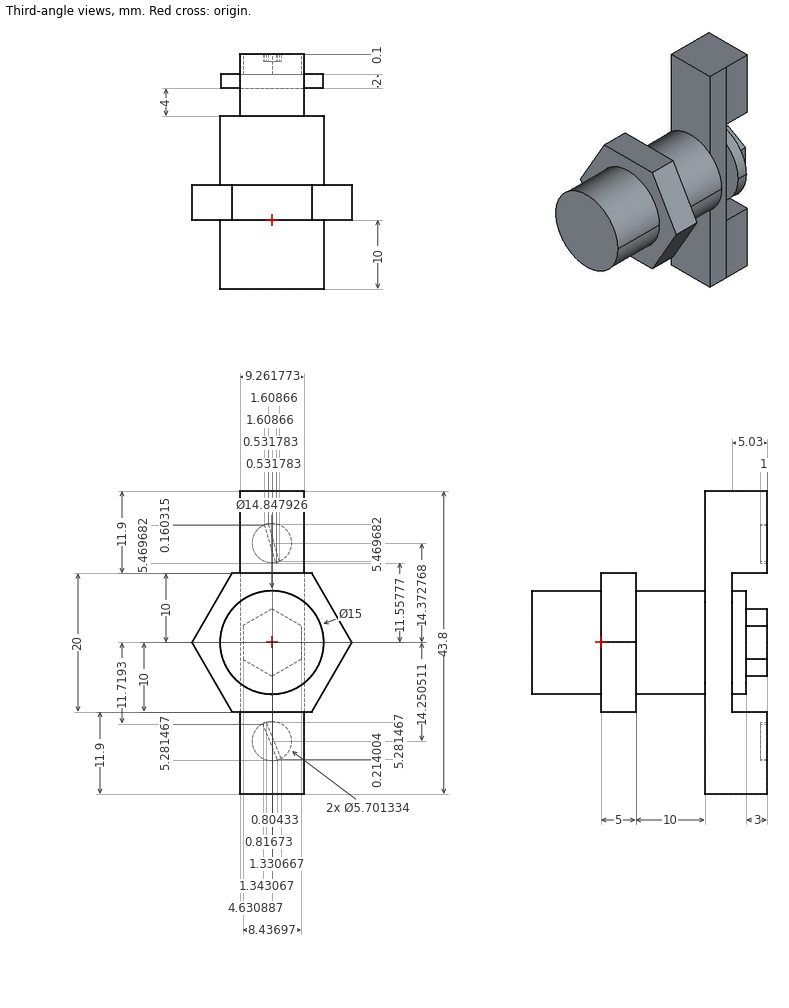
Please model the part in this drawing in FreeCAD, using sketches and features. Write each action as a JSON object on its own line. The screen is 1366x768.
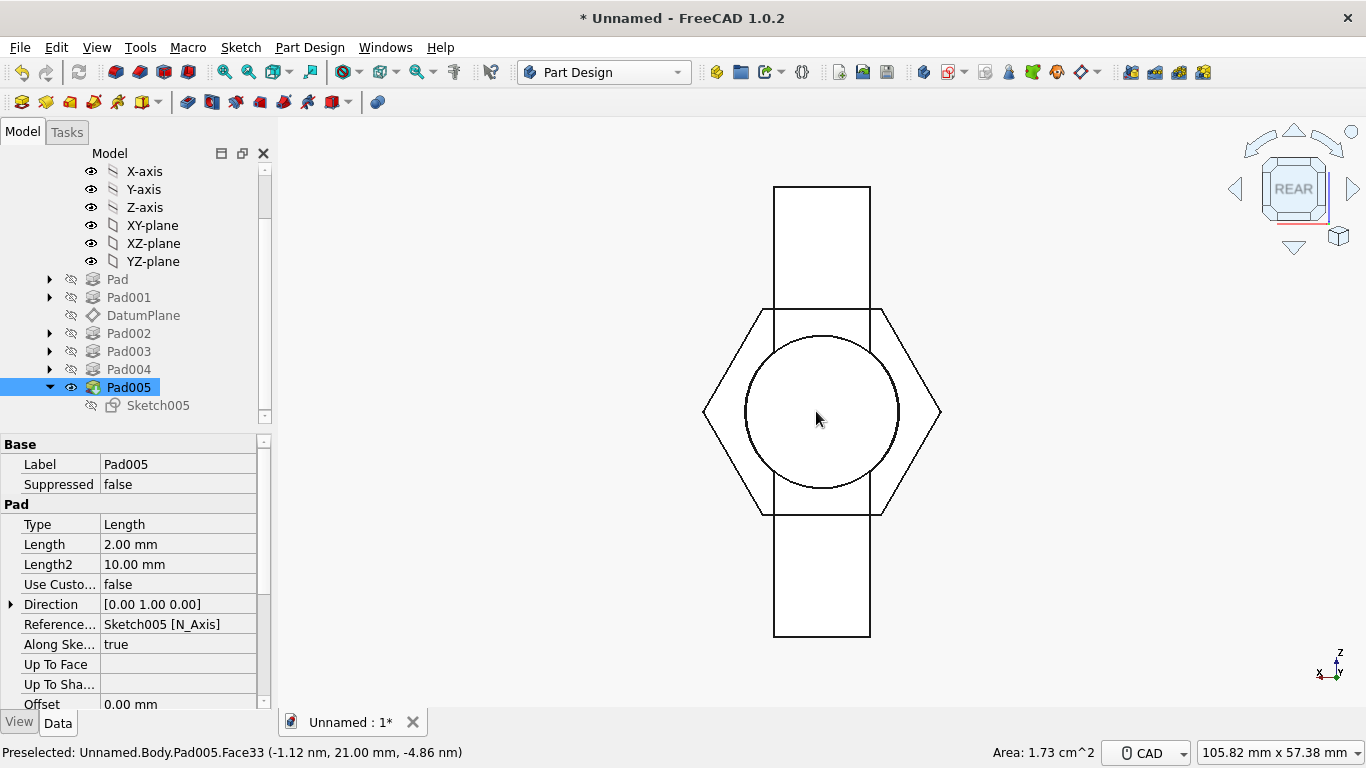
{"action": "left_click", "coordinate": [948, 72]}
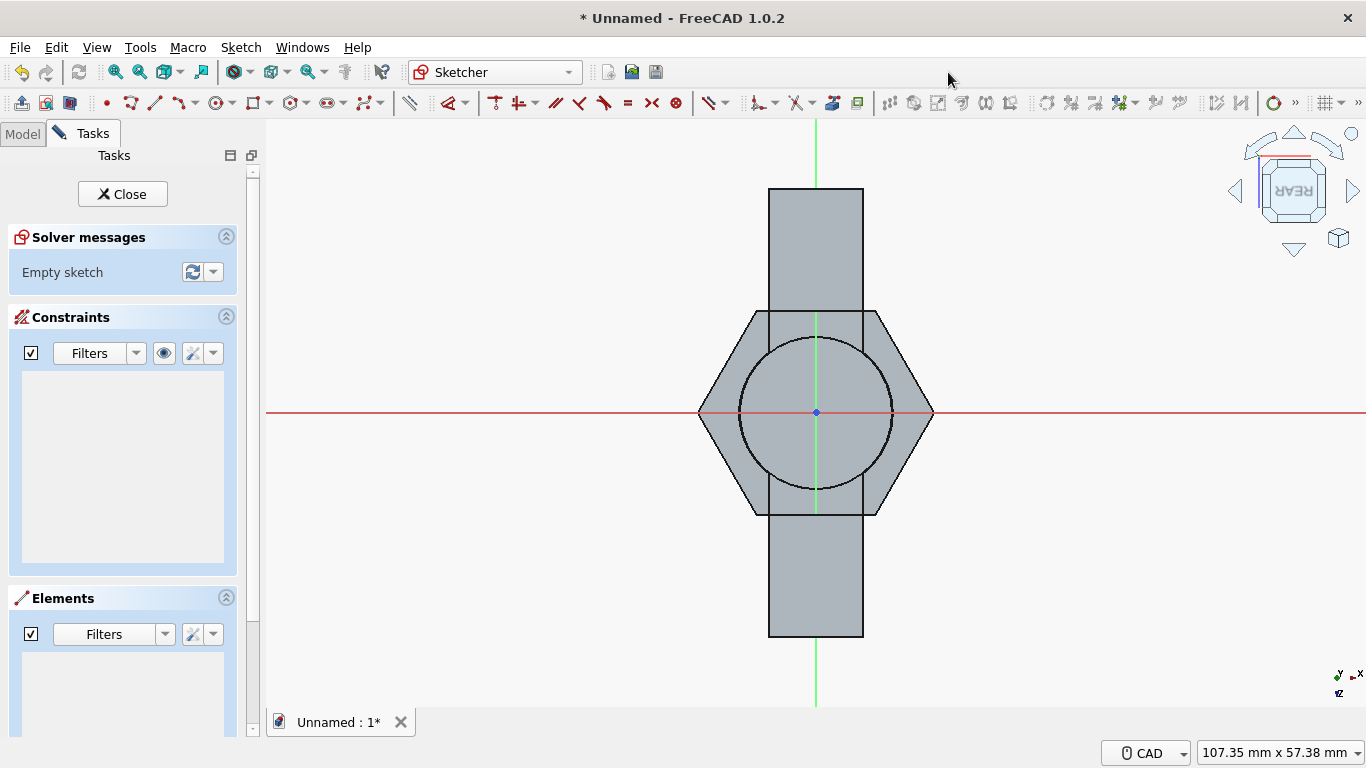
{"action": "scroll", "coordinate": [838, 413], "scroll_direction": "up", "scroll_amount": 7}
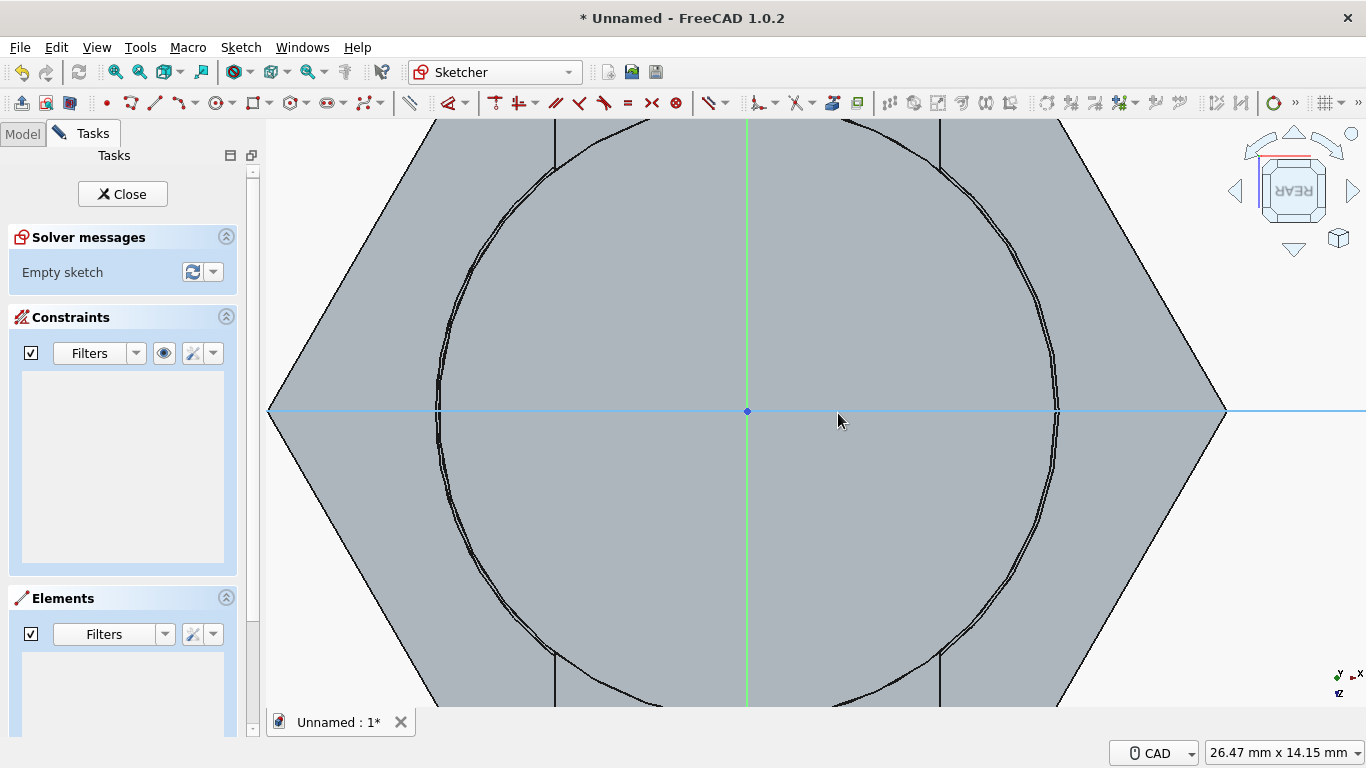
{"action": "left_click", "coordinate": [290, 104]}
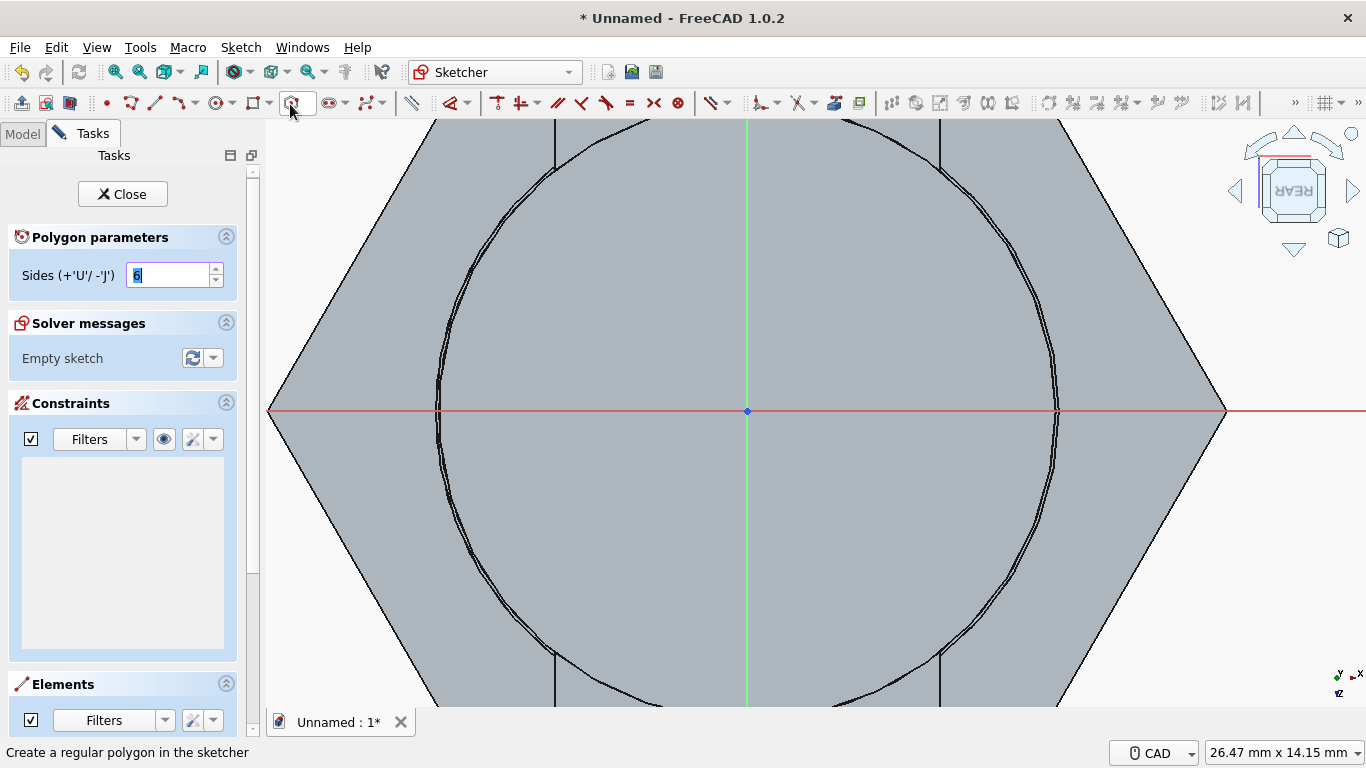
{"action": "left_click", "coordinate": [747, 411]}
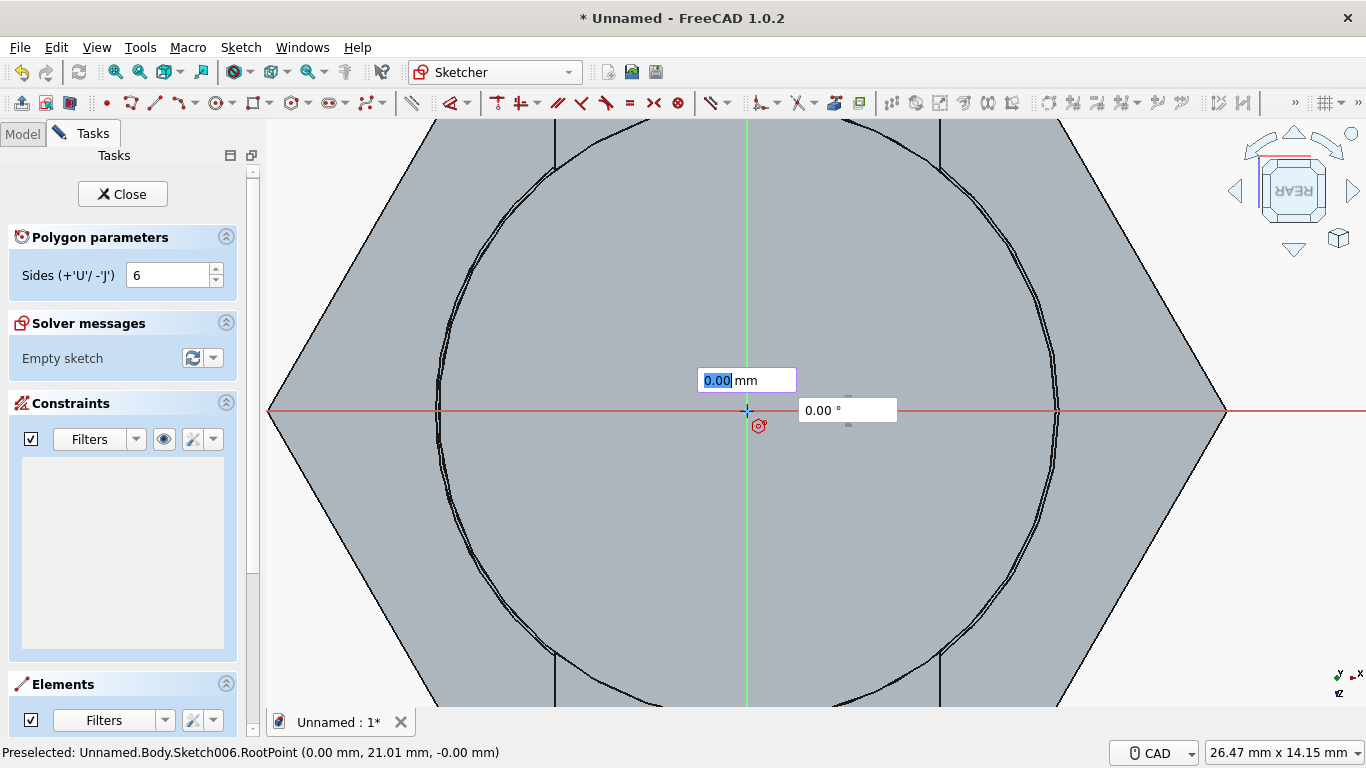
{"action": "left_click", "coordinate": [747, 209]}
{"action": "right_click", "coordinate": [747, 209]}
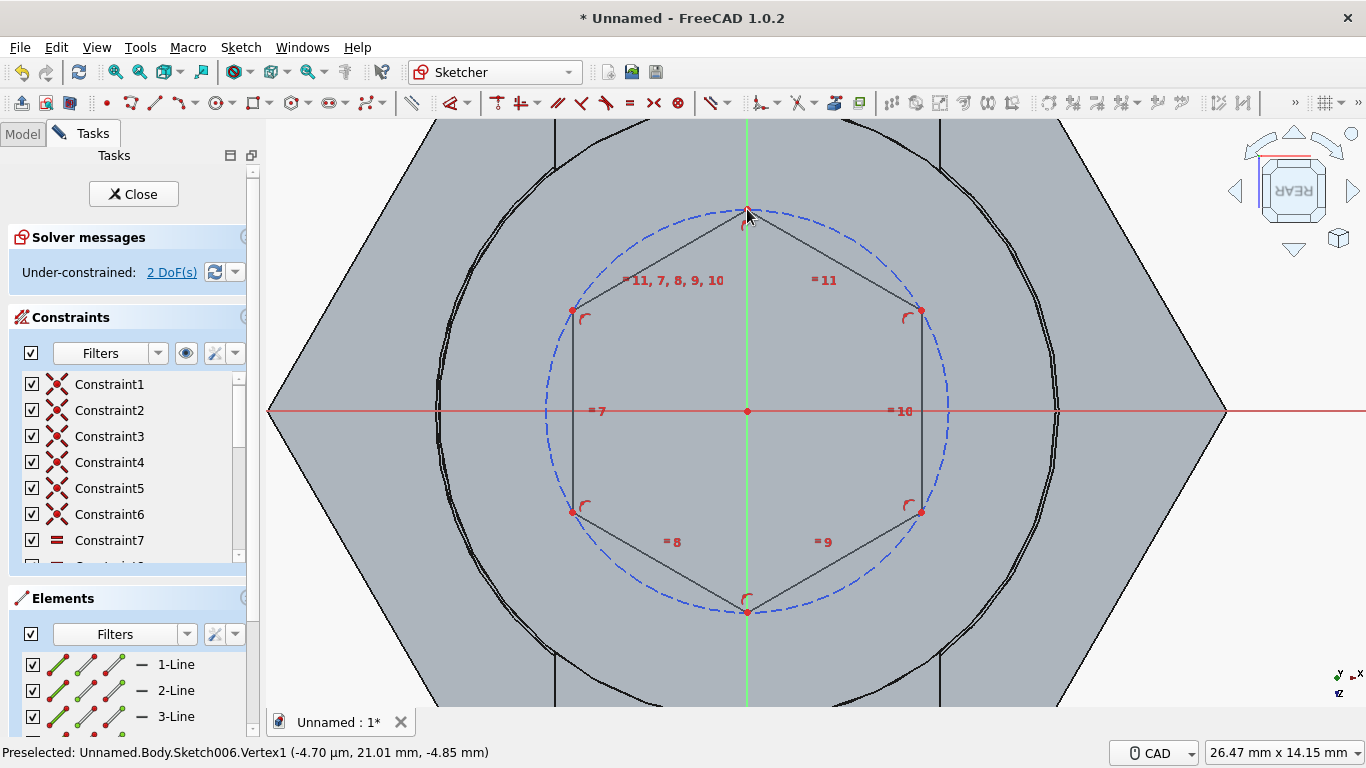
{"action": "left_click", "coordinate": [573, 371]}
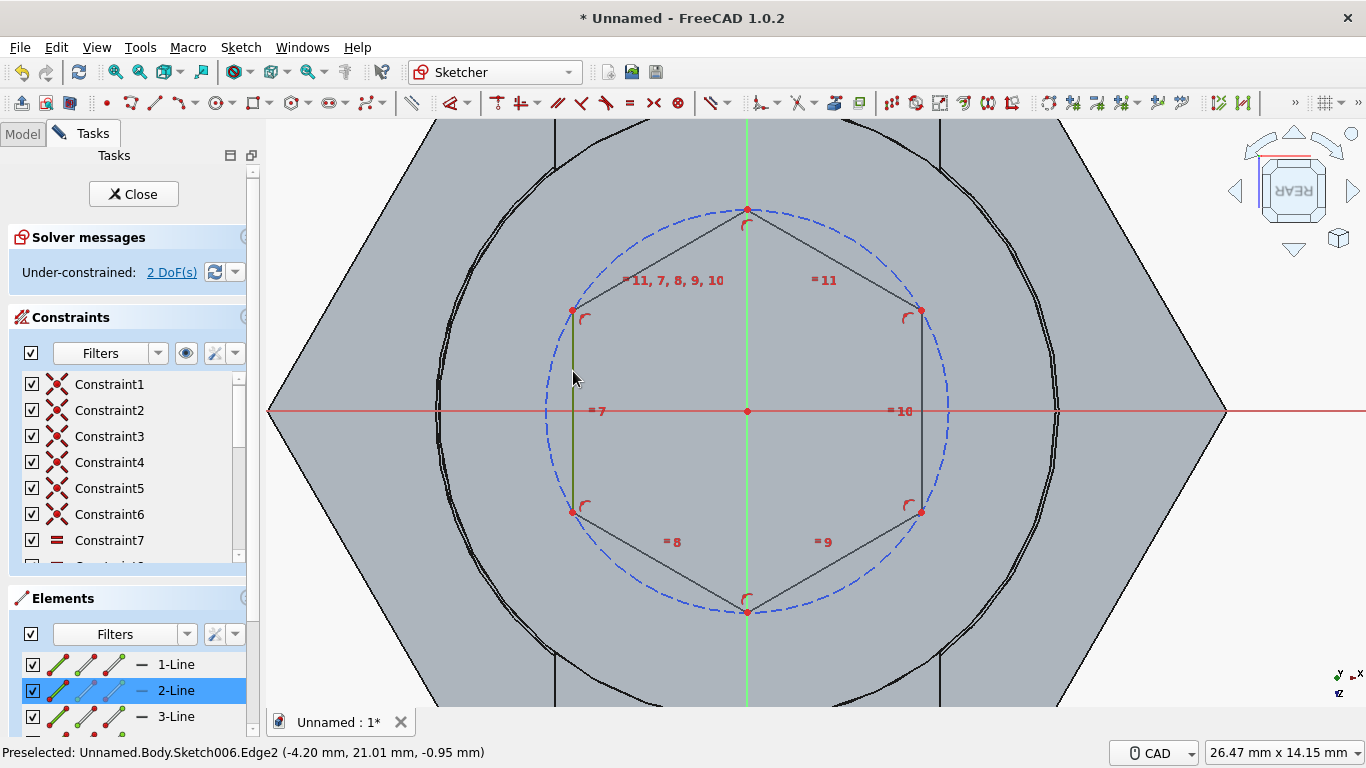
{"action": "key", "text": "v"}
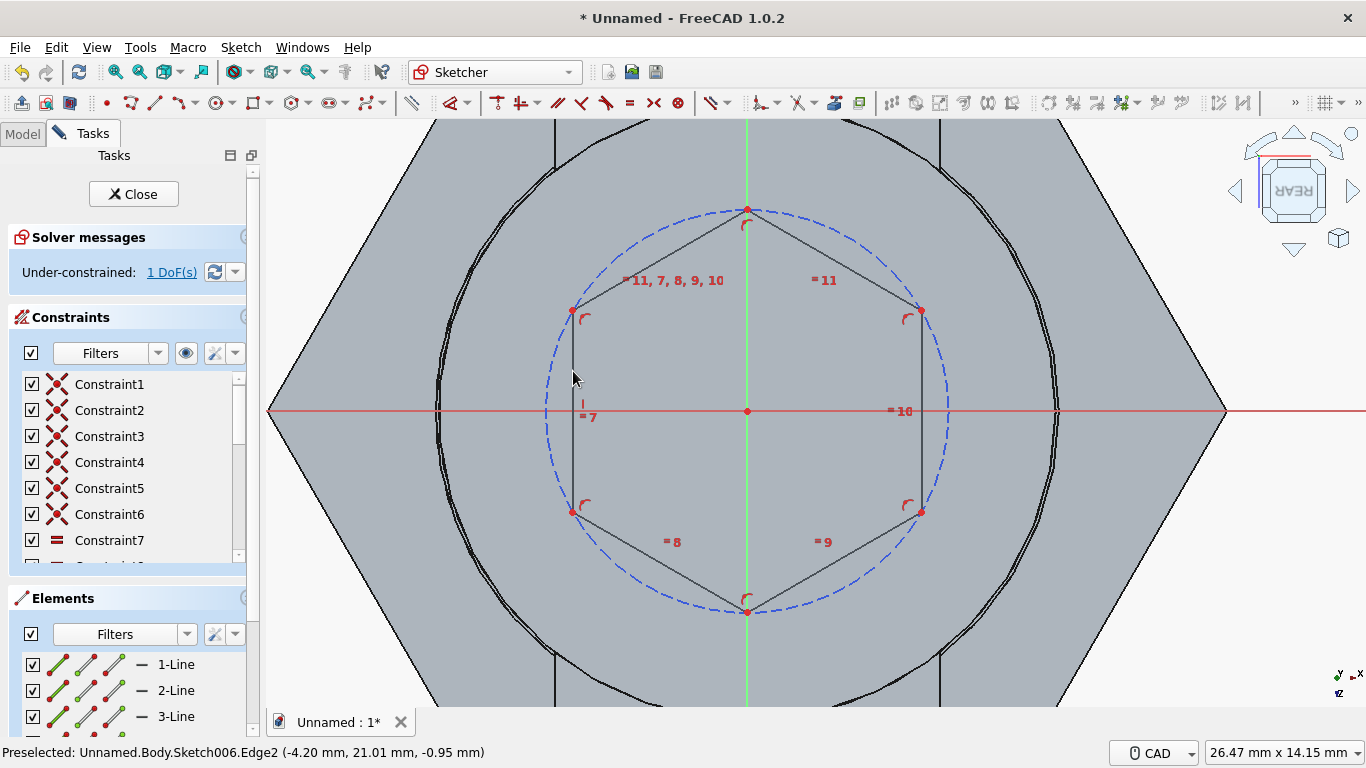
{"action": "left_click", "coordinate": [450, 104]}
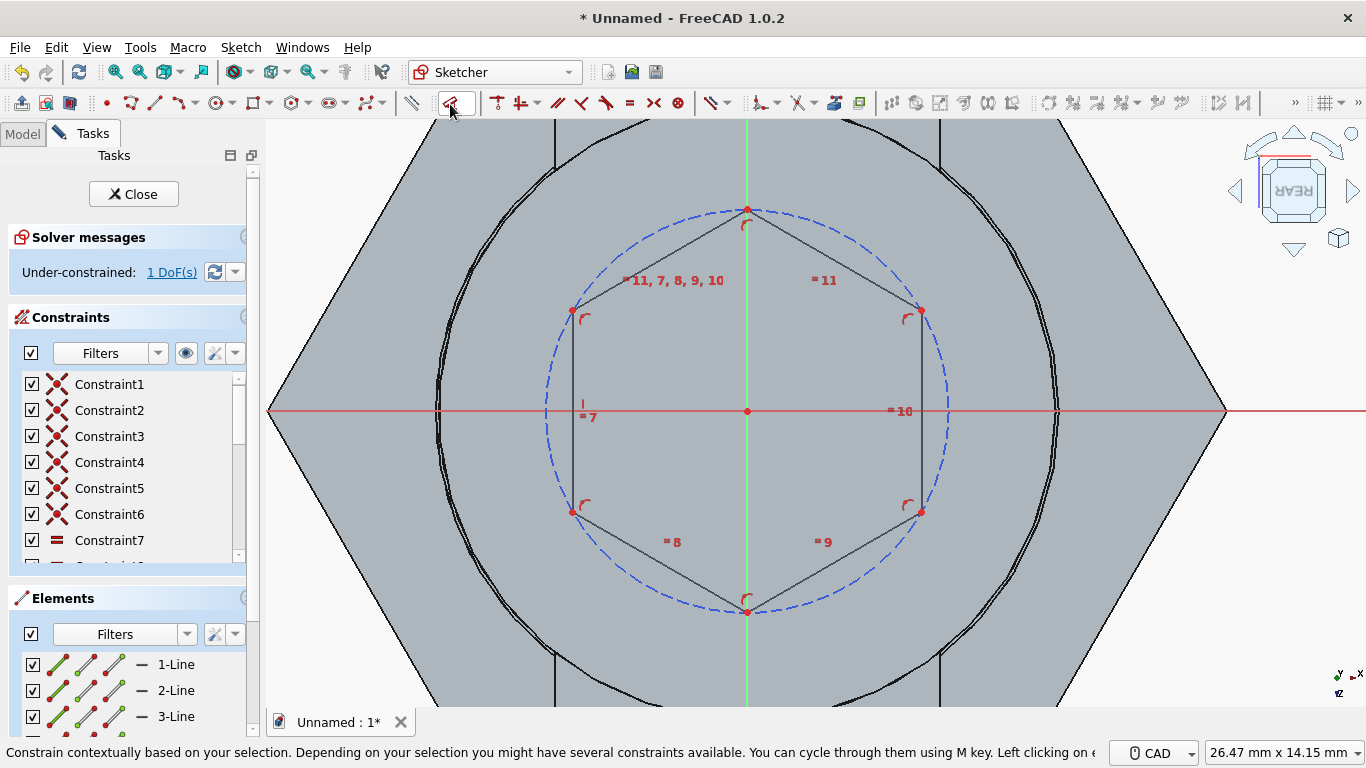
{"action": "left_click", "coordinate": [573, 311]}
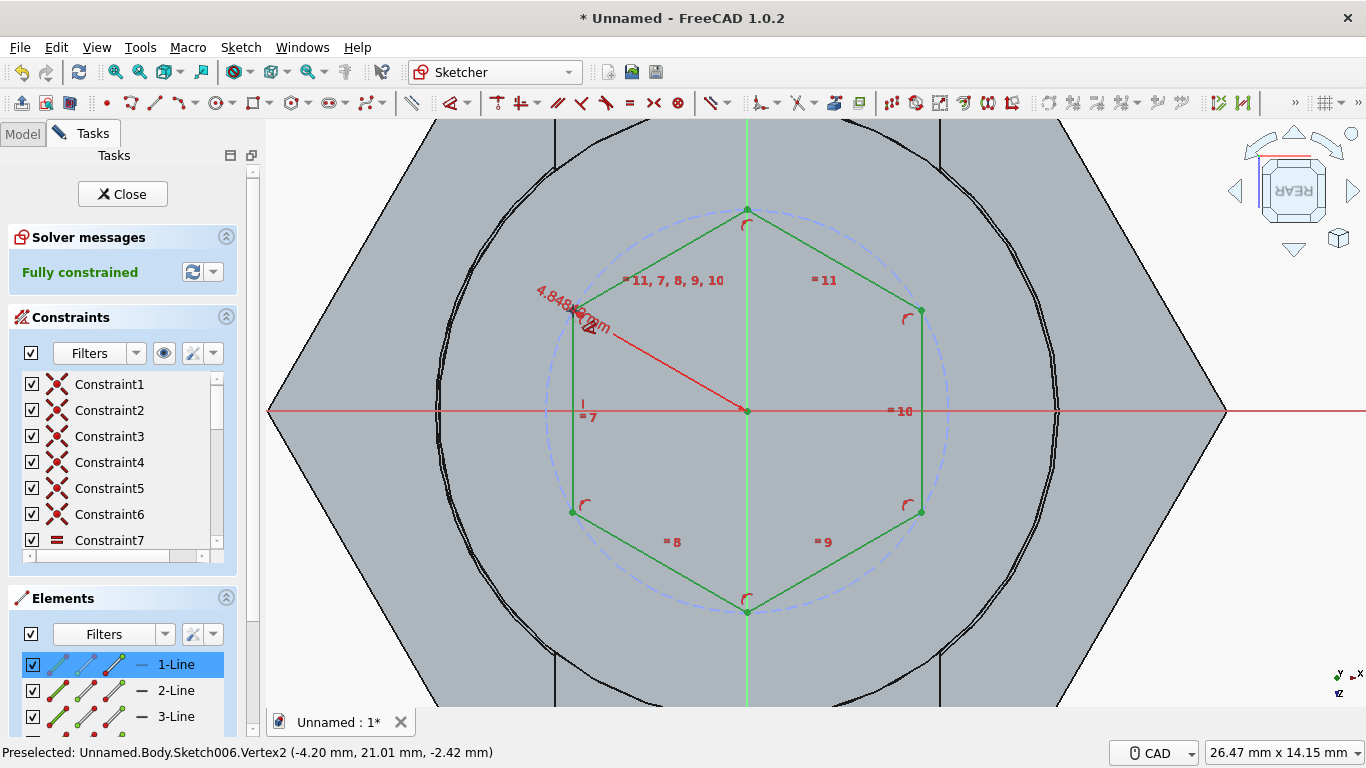
{"action": "left_click", "coordinate": [922, 512]}
{"action": "left_click", "coordinate": [667, 277]}